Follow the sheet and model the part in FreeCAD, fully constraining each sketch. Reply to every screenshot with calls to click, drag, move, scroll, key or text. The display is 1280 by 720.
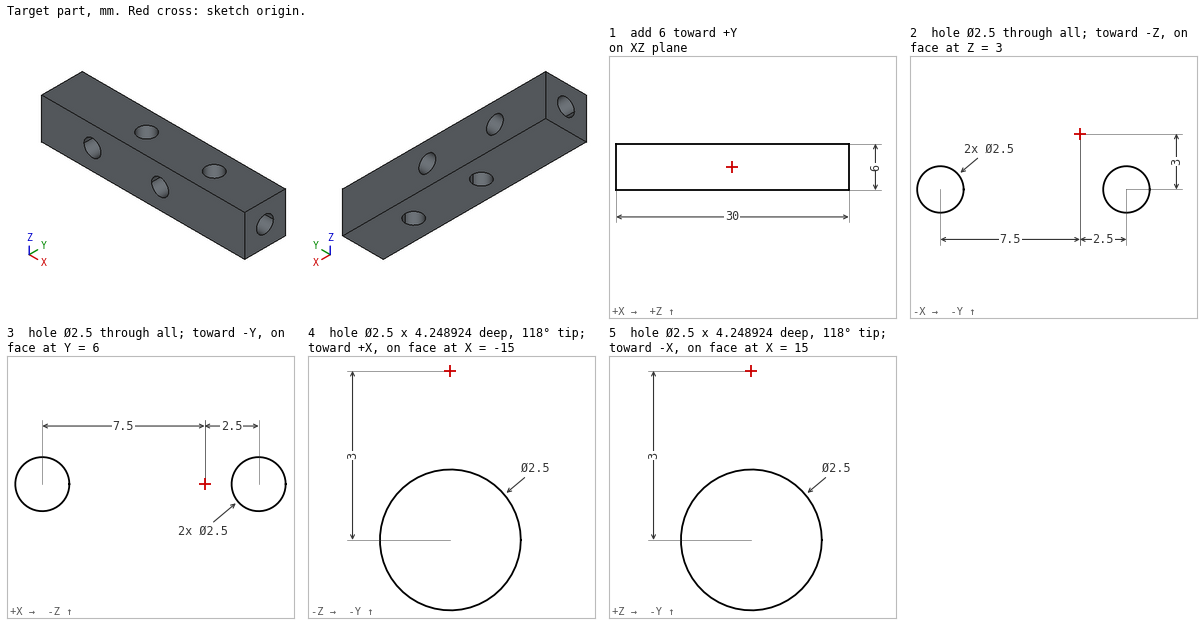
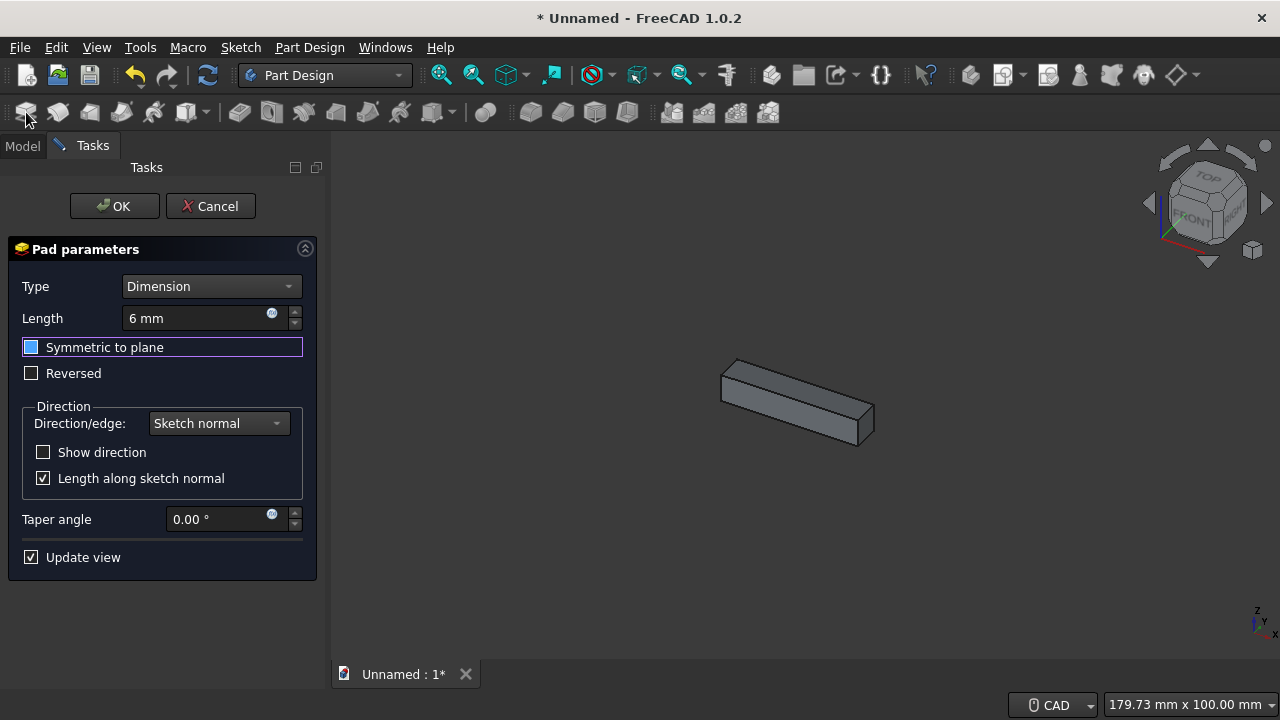
click(30, 373)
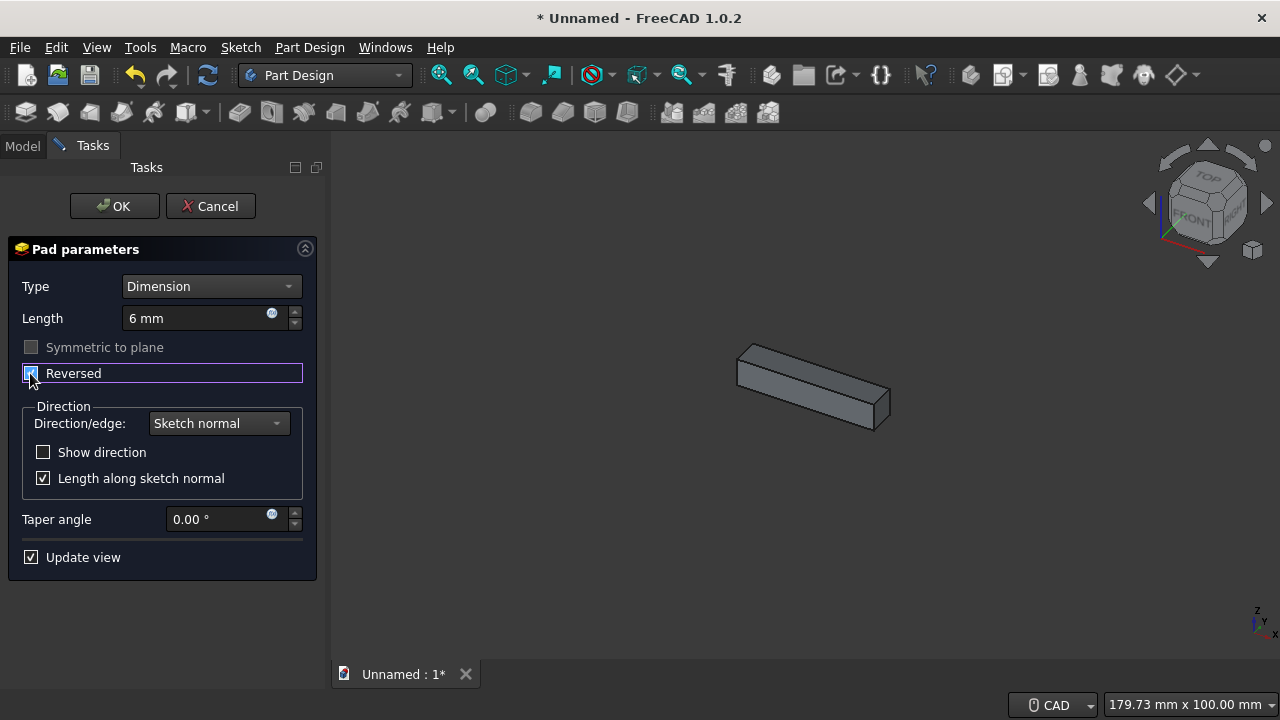
click(115, 206)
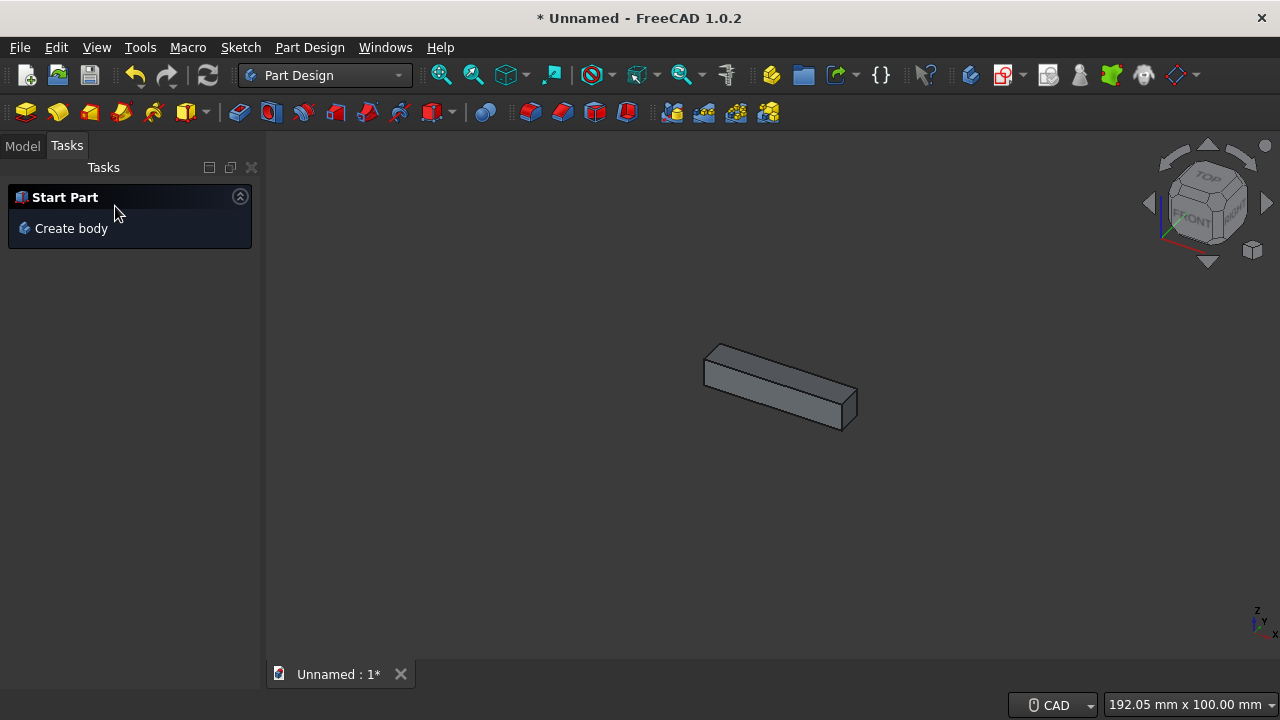
key(v)
key(f)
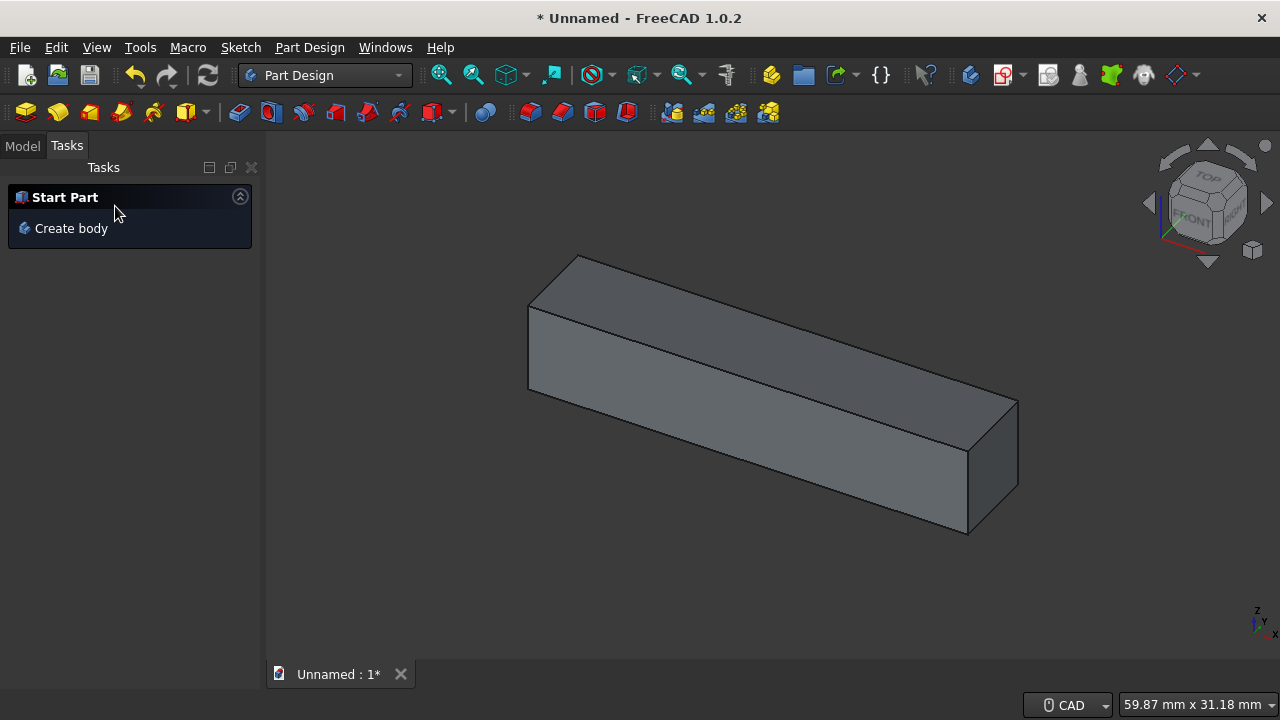
click(899, 394)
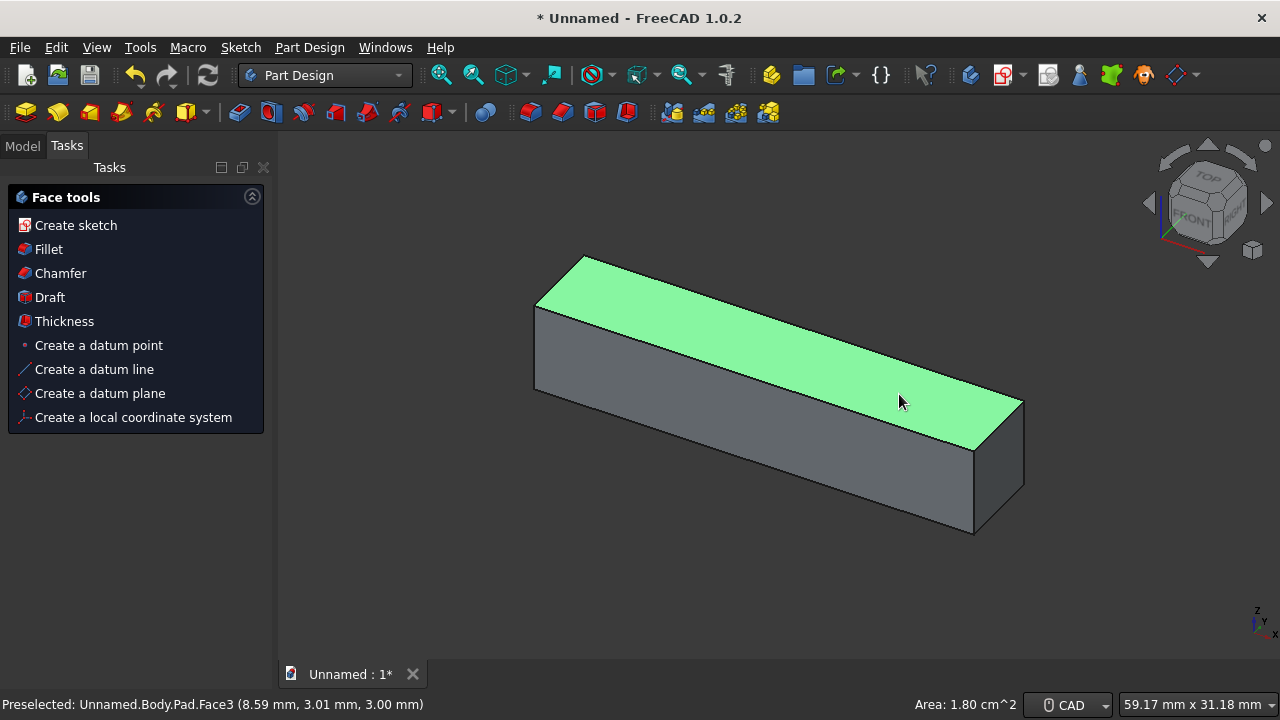
click(1004, 76)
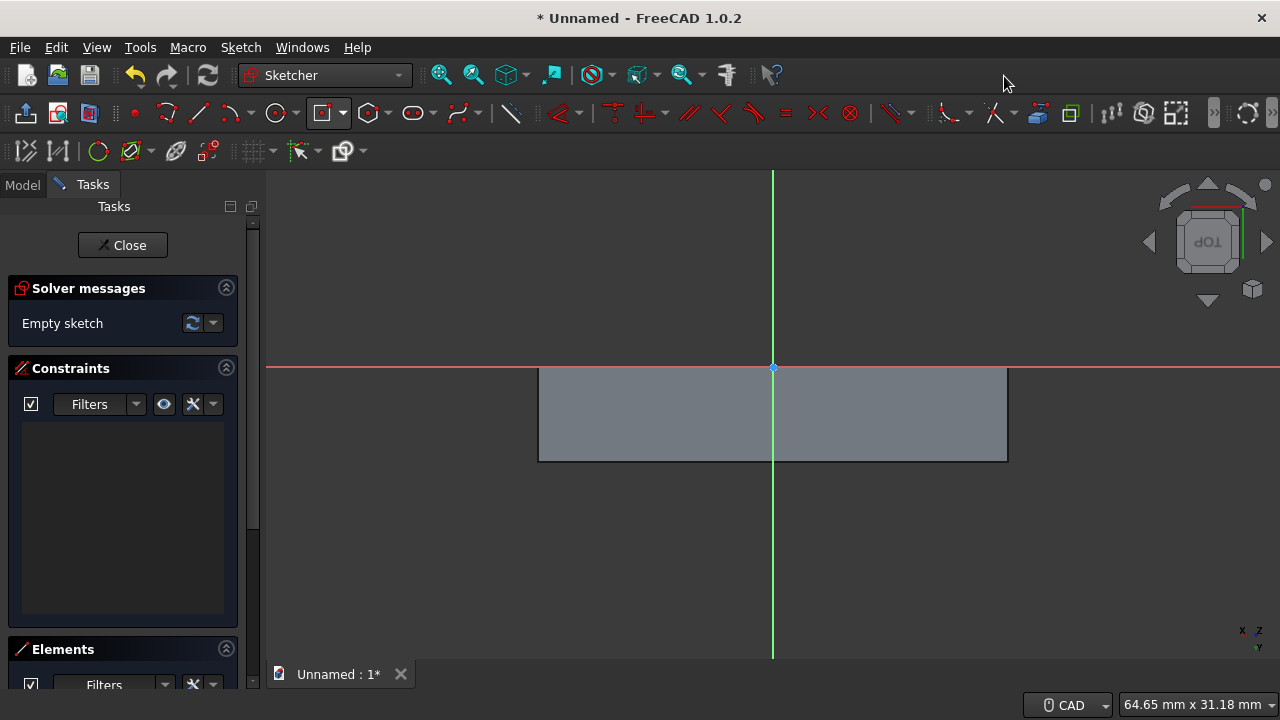
scroll(751, 393, up, 5)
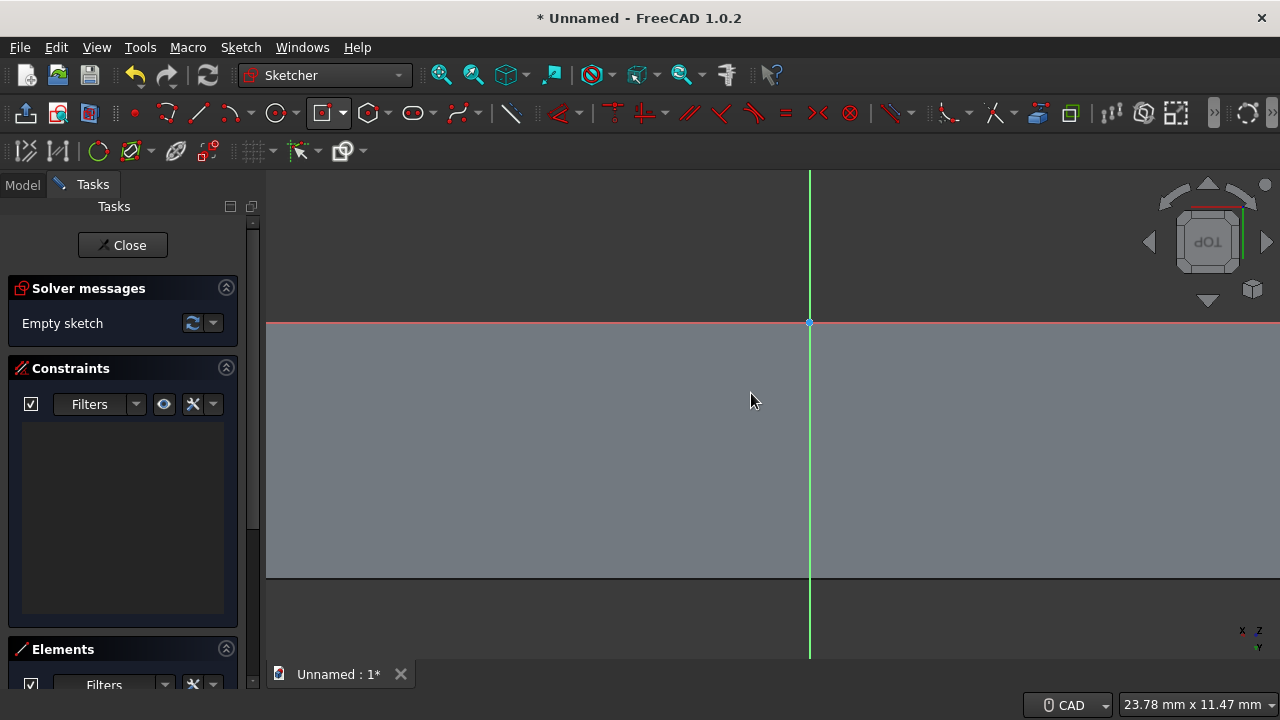
key(g)
key(c)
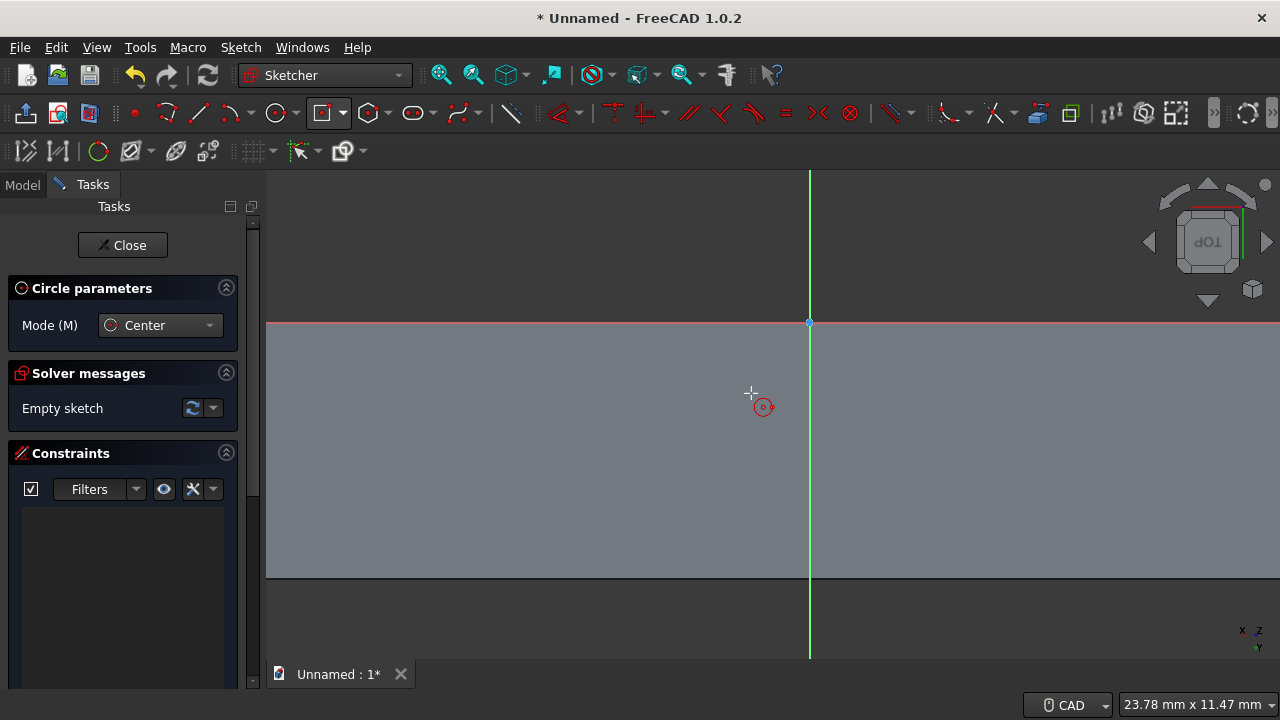
click(917, 451)
move(954, 413)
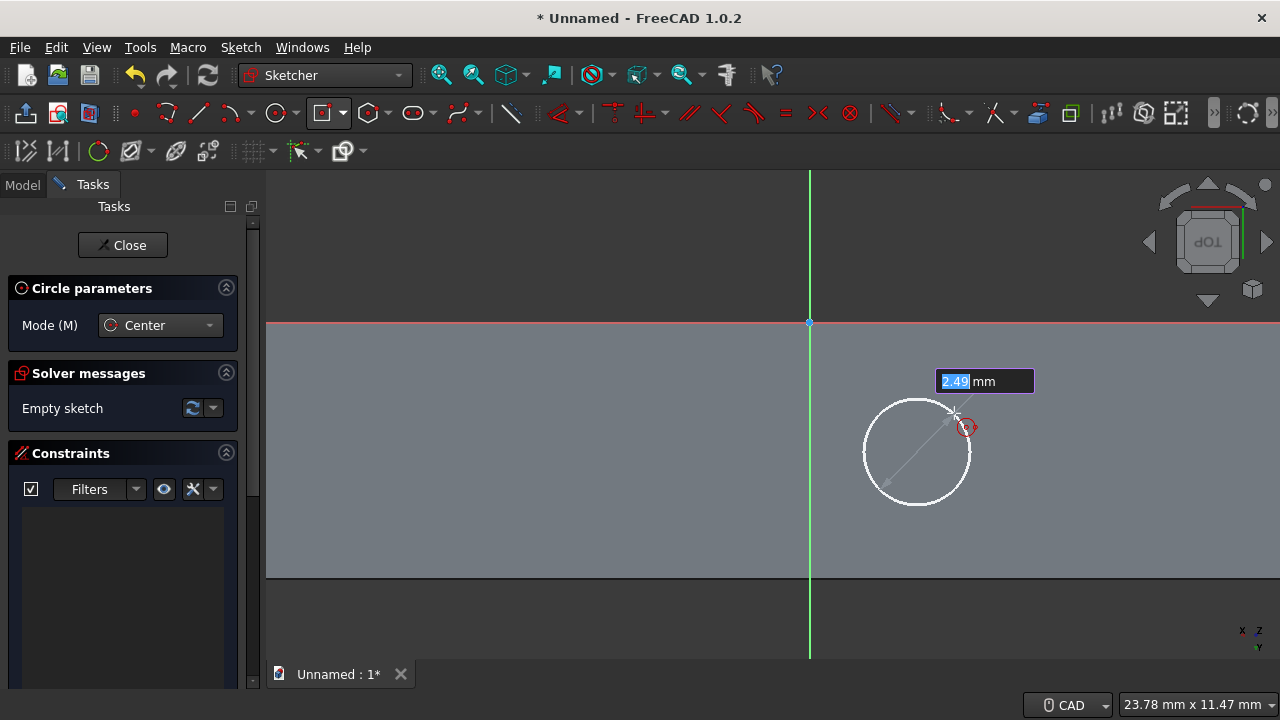
text(2.5)
key(Return)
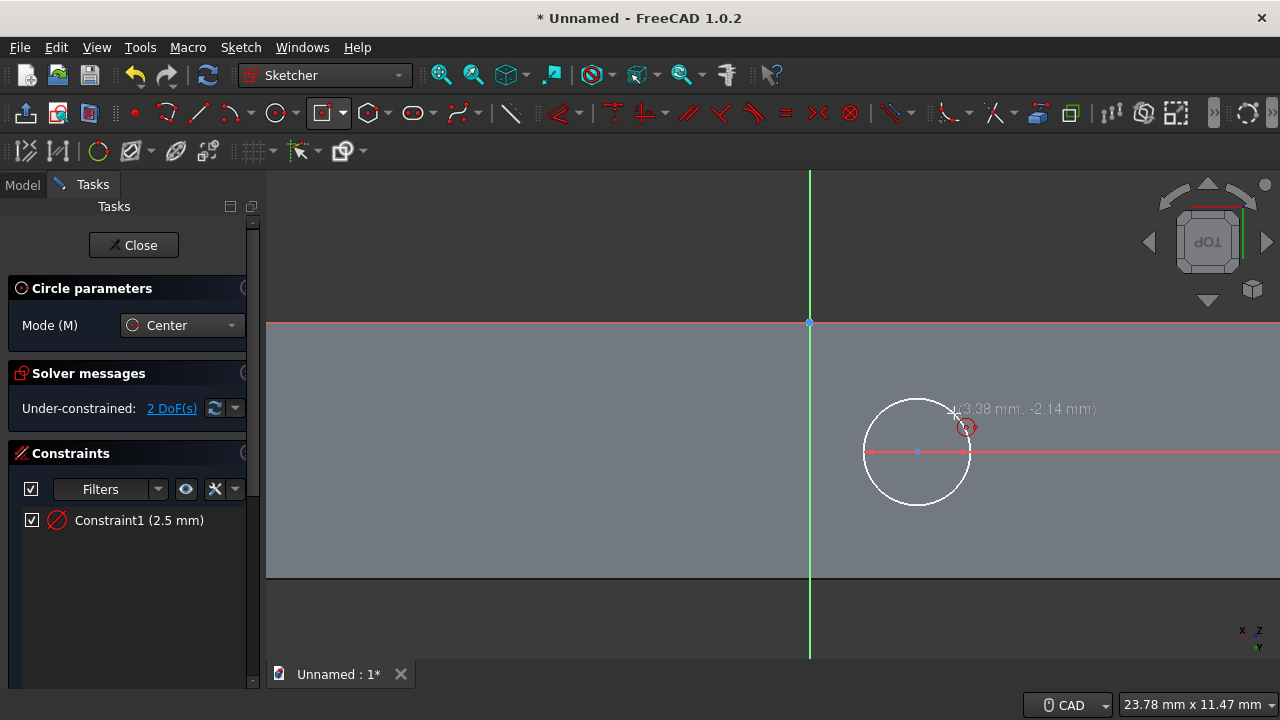
click(490, 451)
move(528, 413)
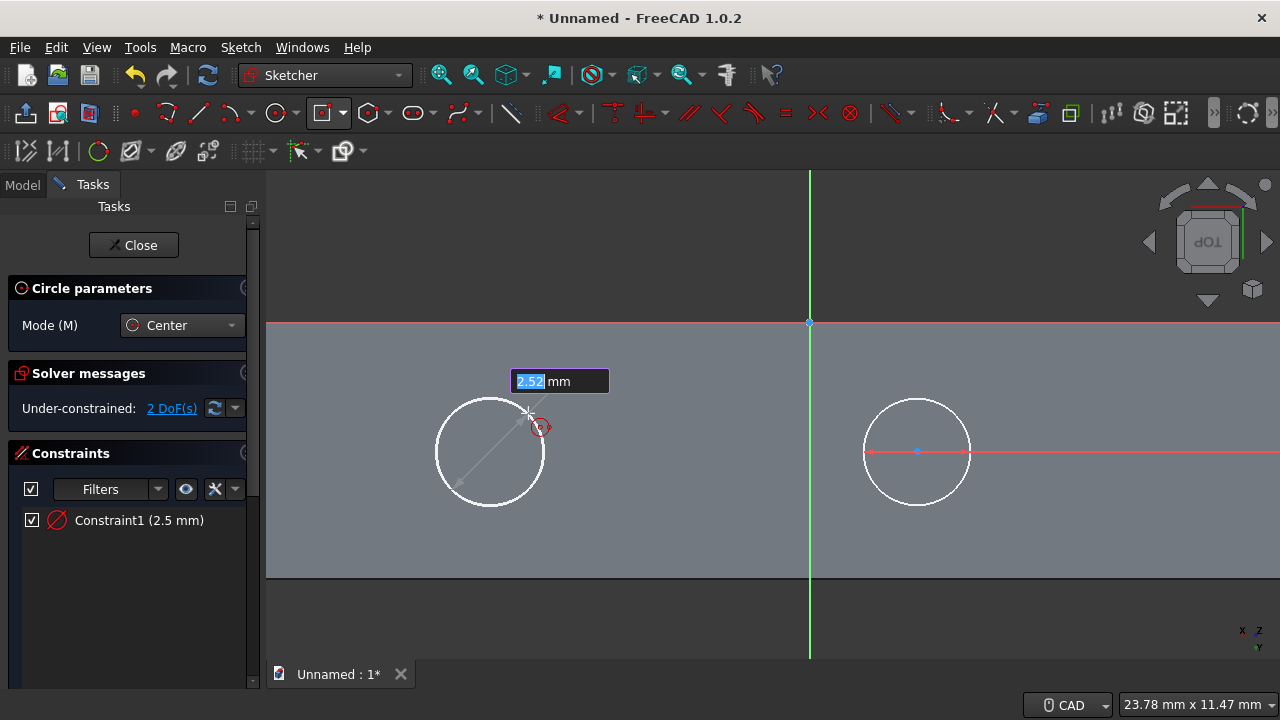
text(2.5)
key(Return)
key(Escape)